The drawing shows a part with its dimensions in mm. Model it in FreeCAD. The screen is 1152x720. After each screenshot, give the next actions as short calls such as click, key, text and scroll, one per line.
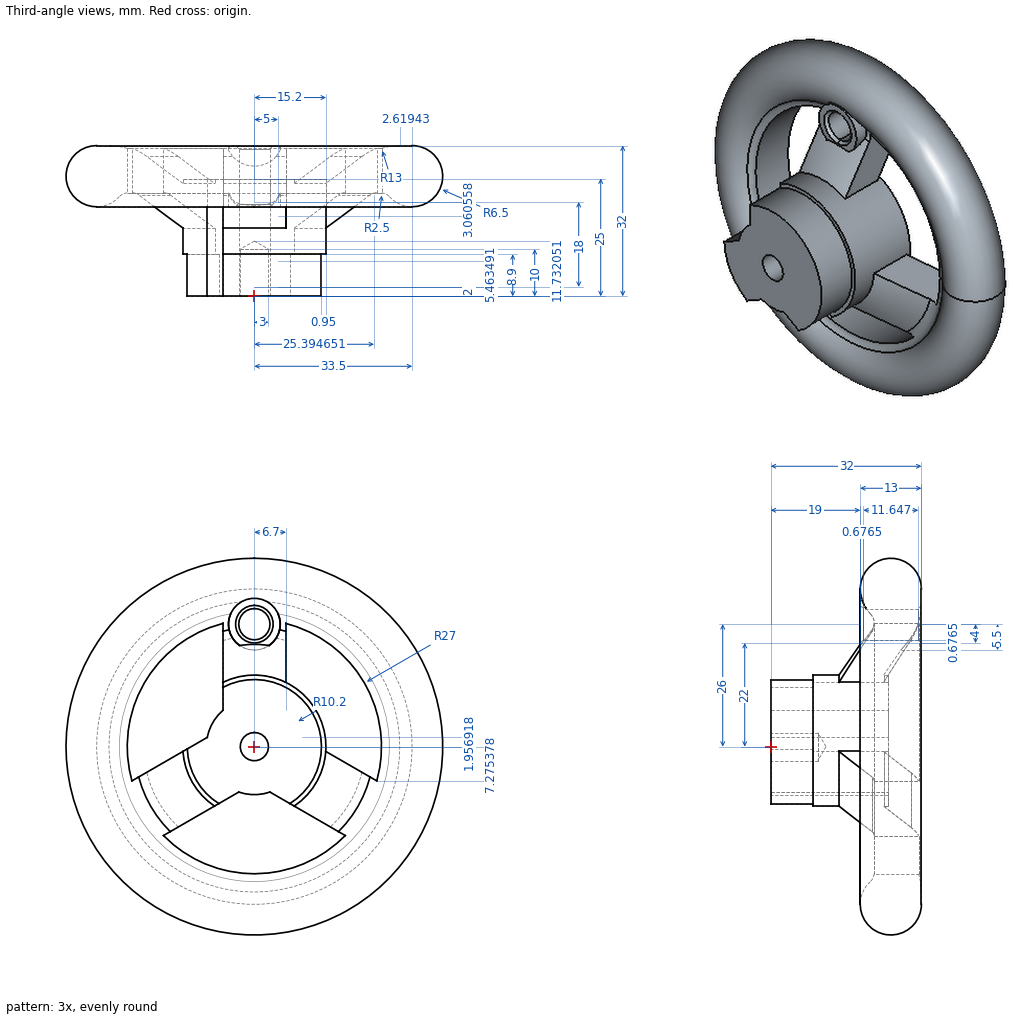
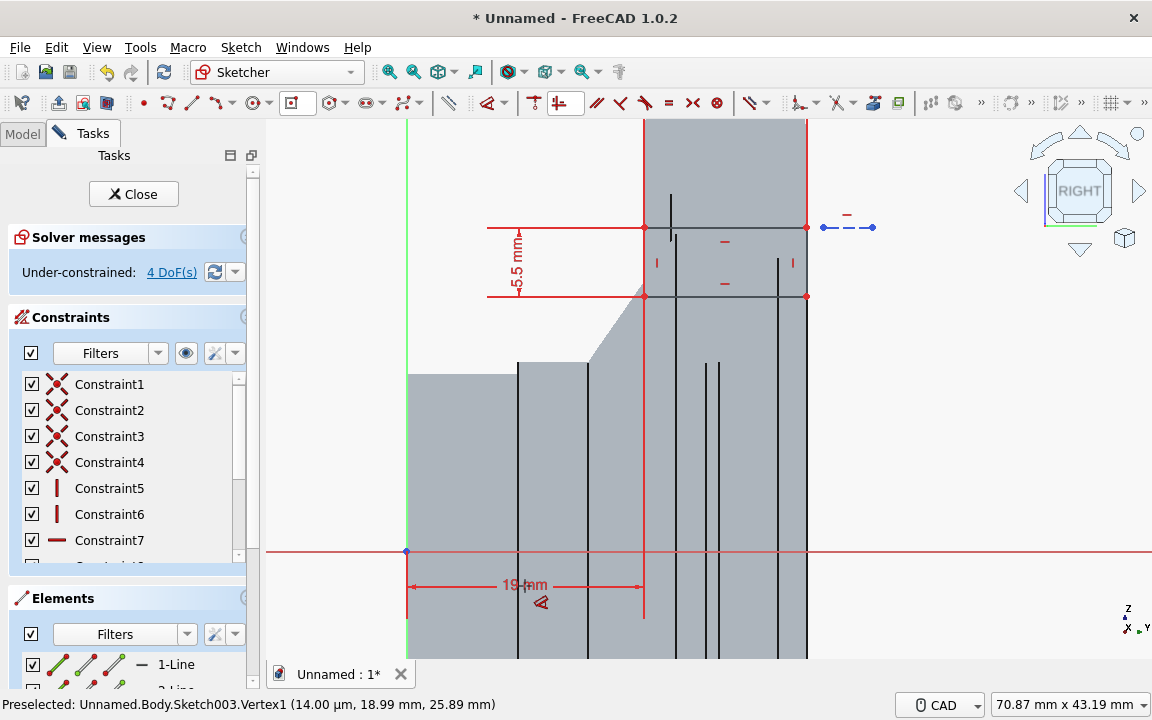
click(644, 228)
click(373, 390)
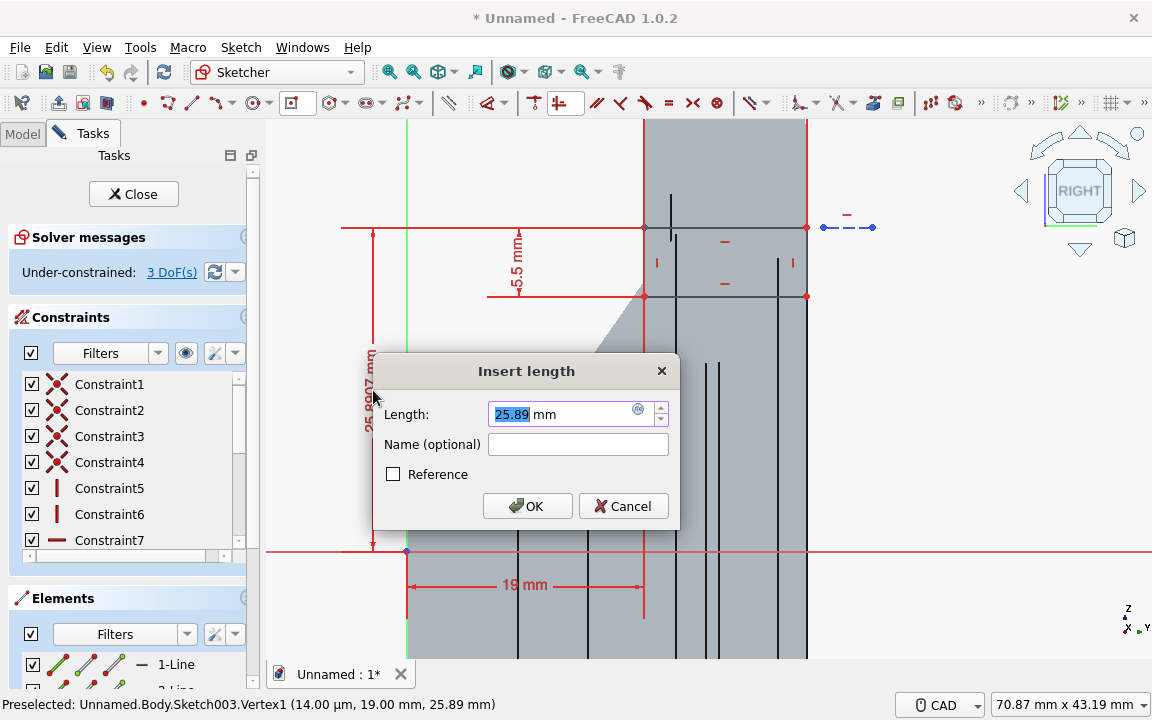
text(26)
key(Return)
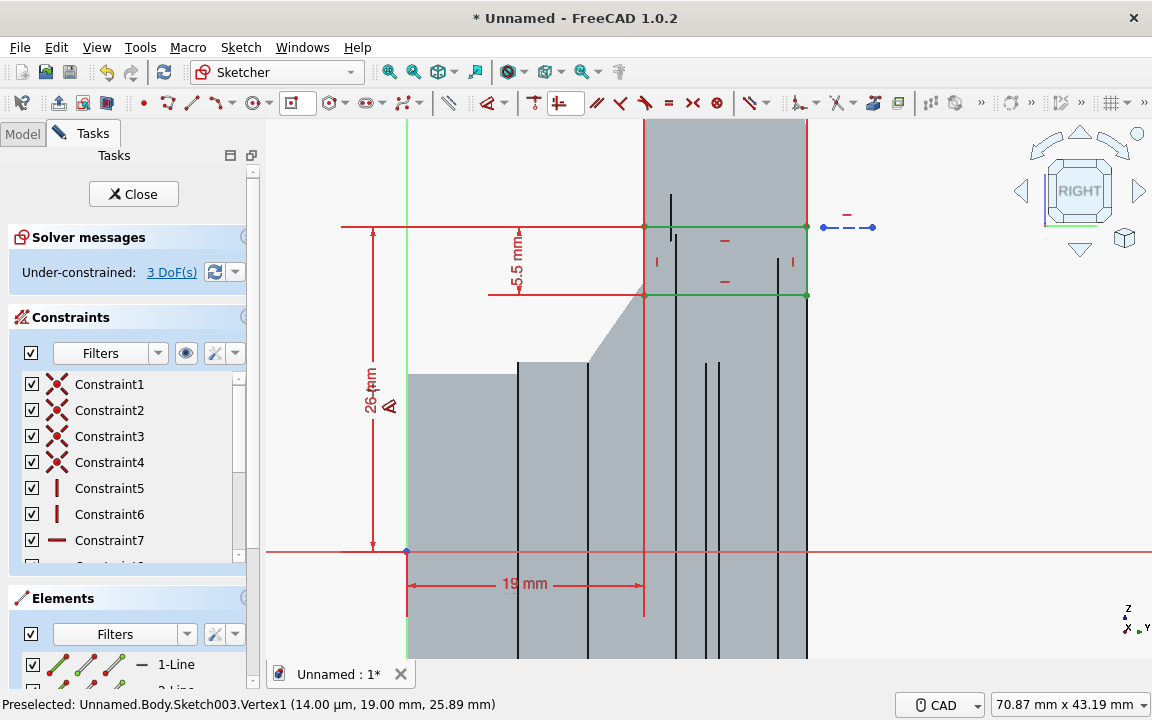
click(823, 228)
click(373, 315)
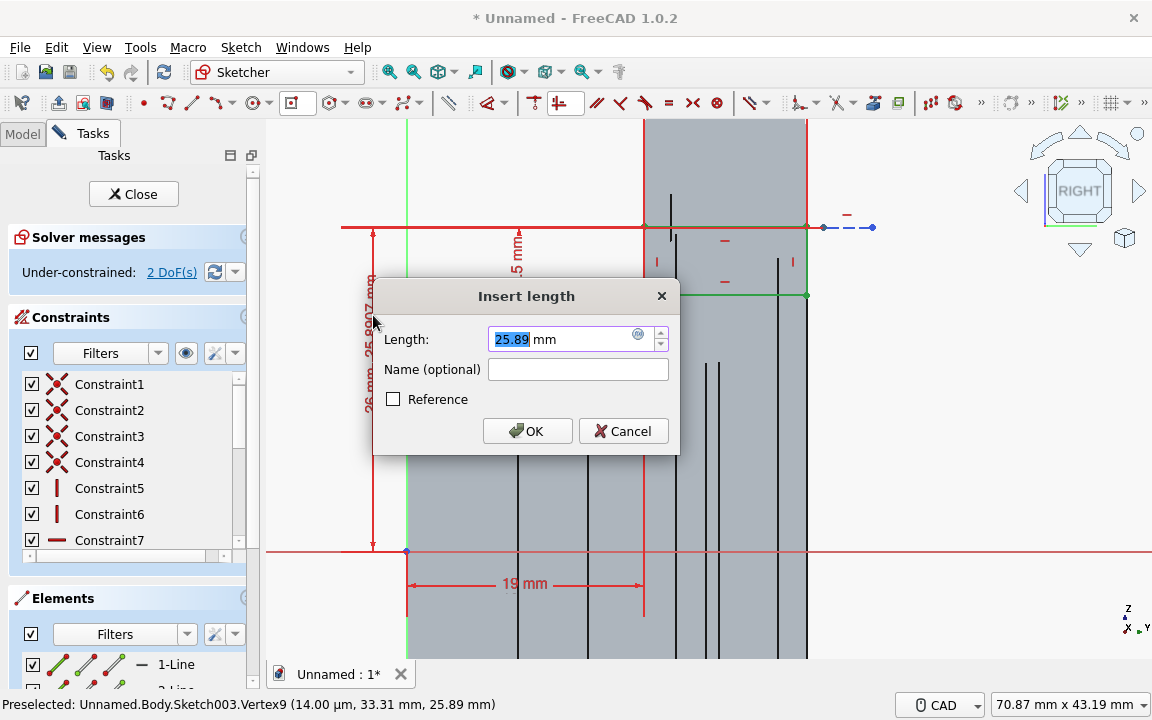
text(26)
key(Return)
key(Escape)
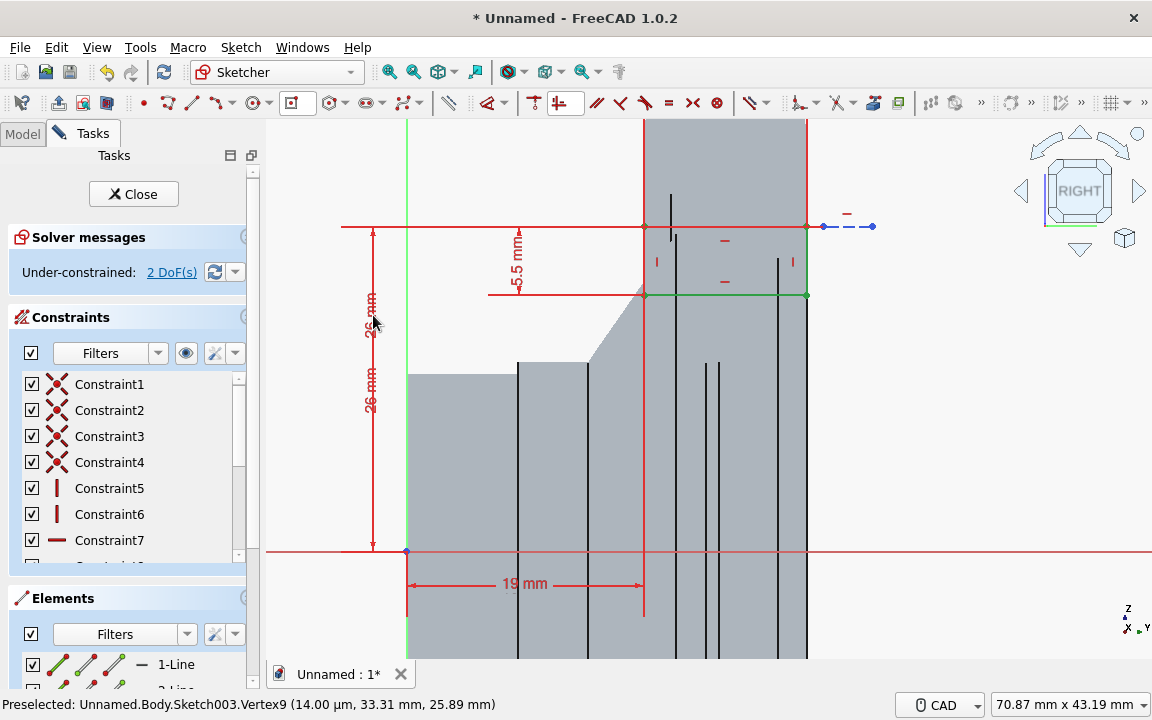
click(134, 194)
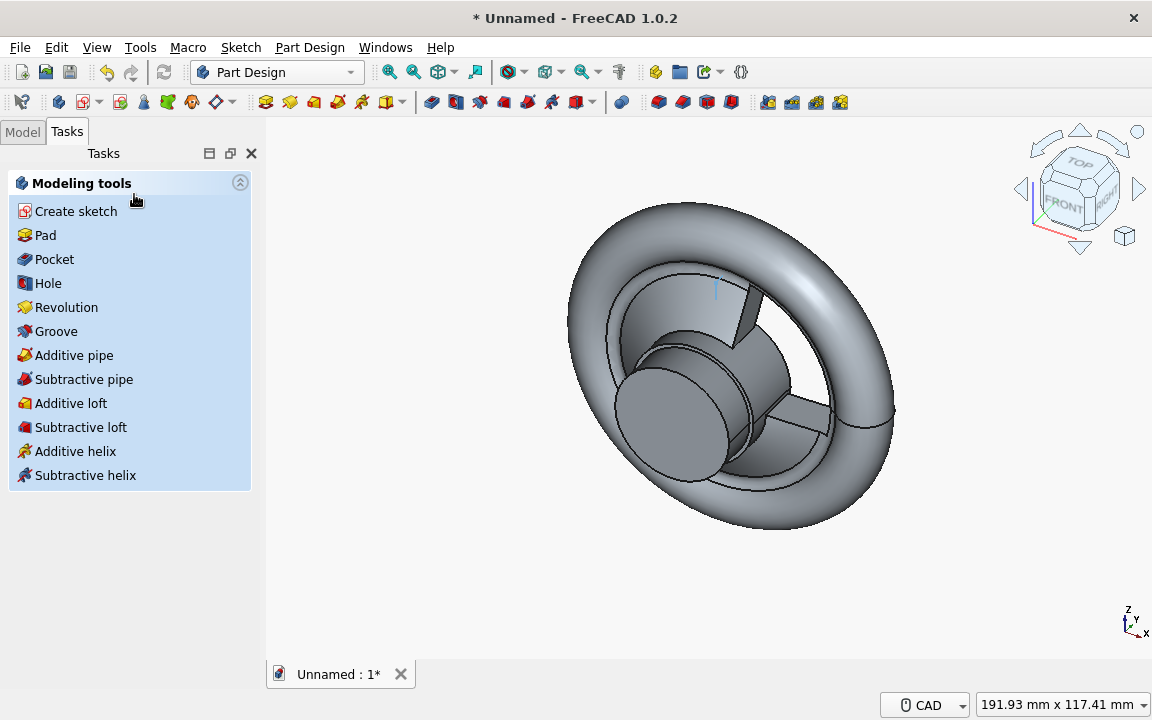
click(290, 102)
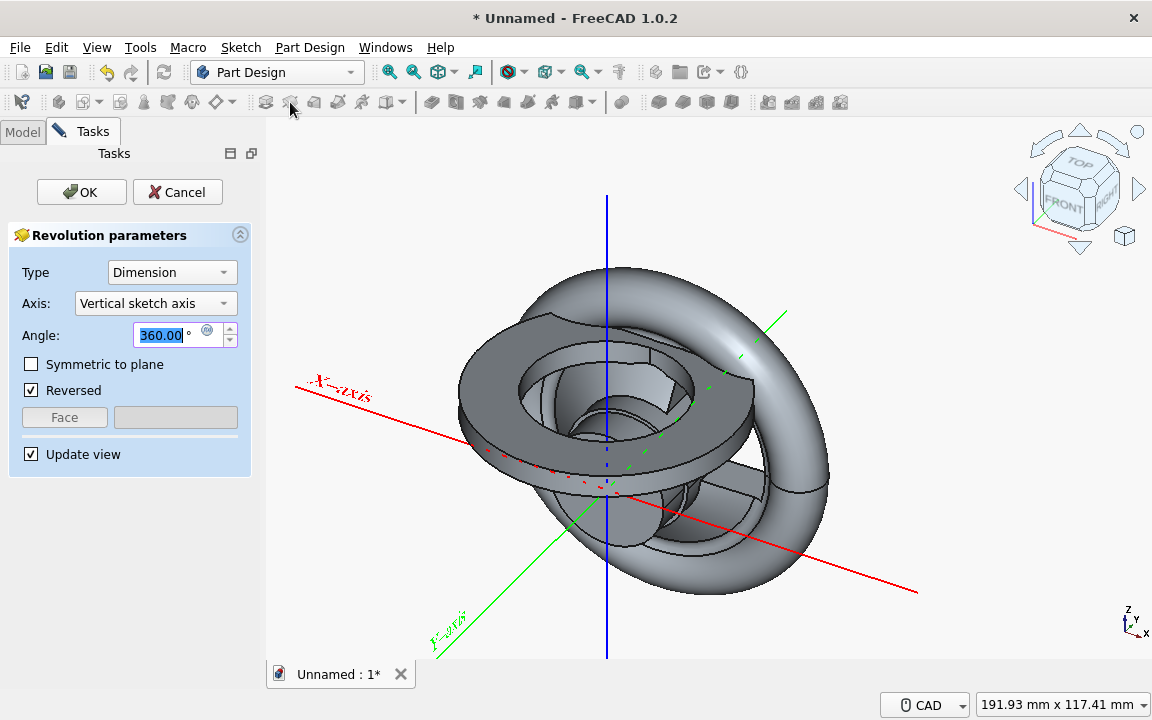
click(156, 304)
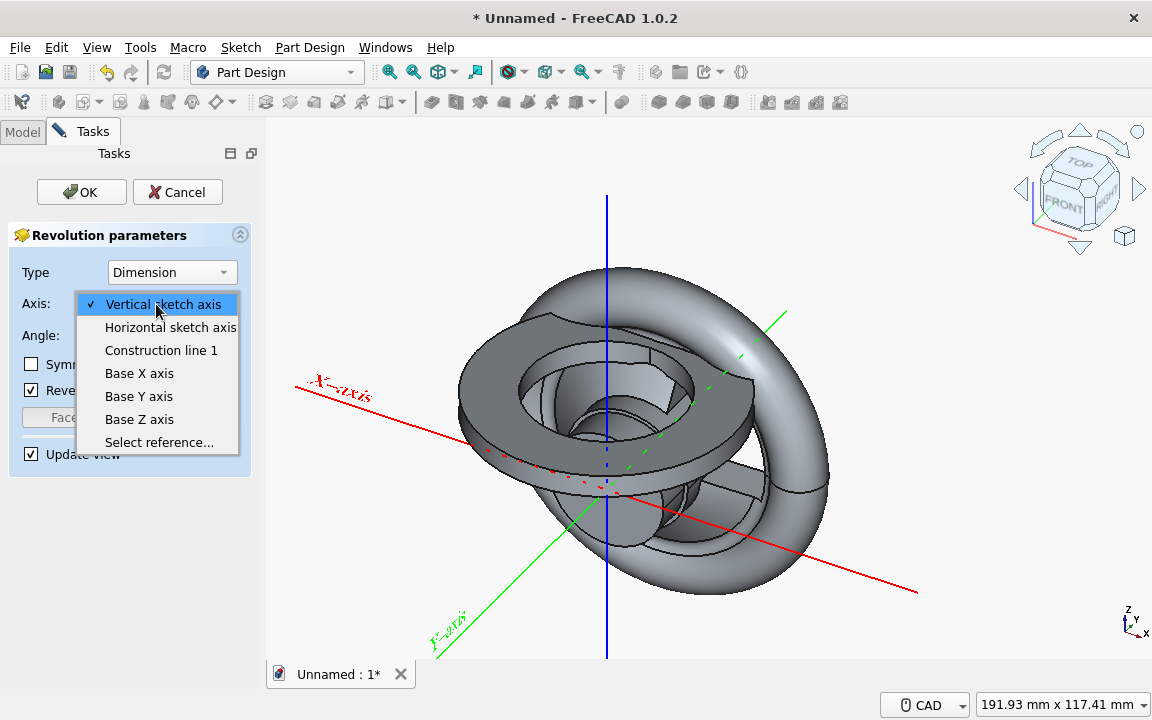
click(156, 350)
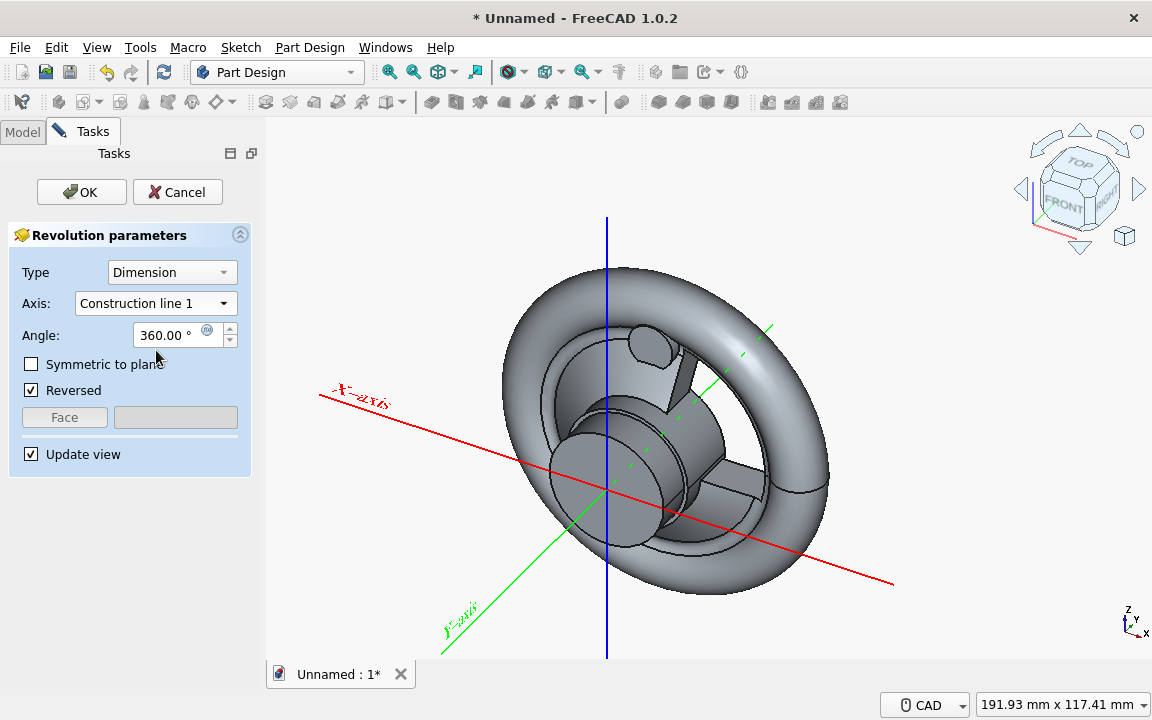
click(82, 192)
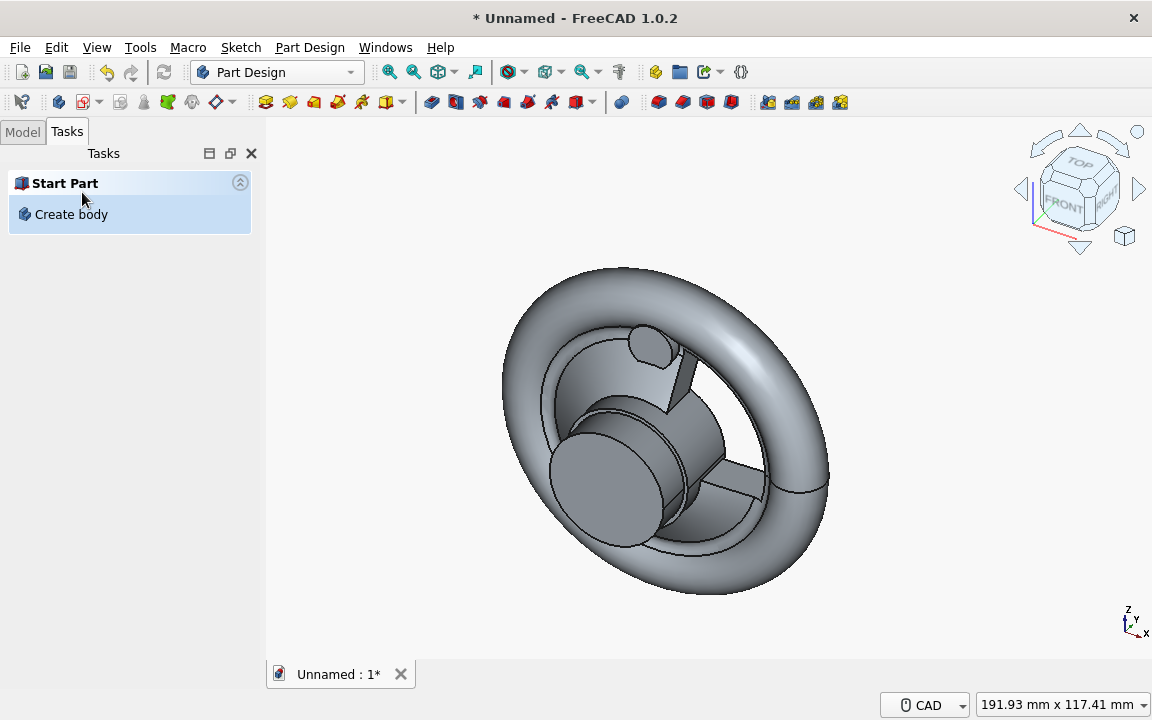
click(390, 72)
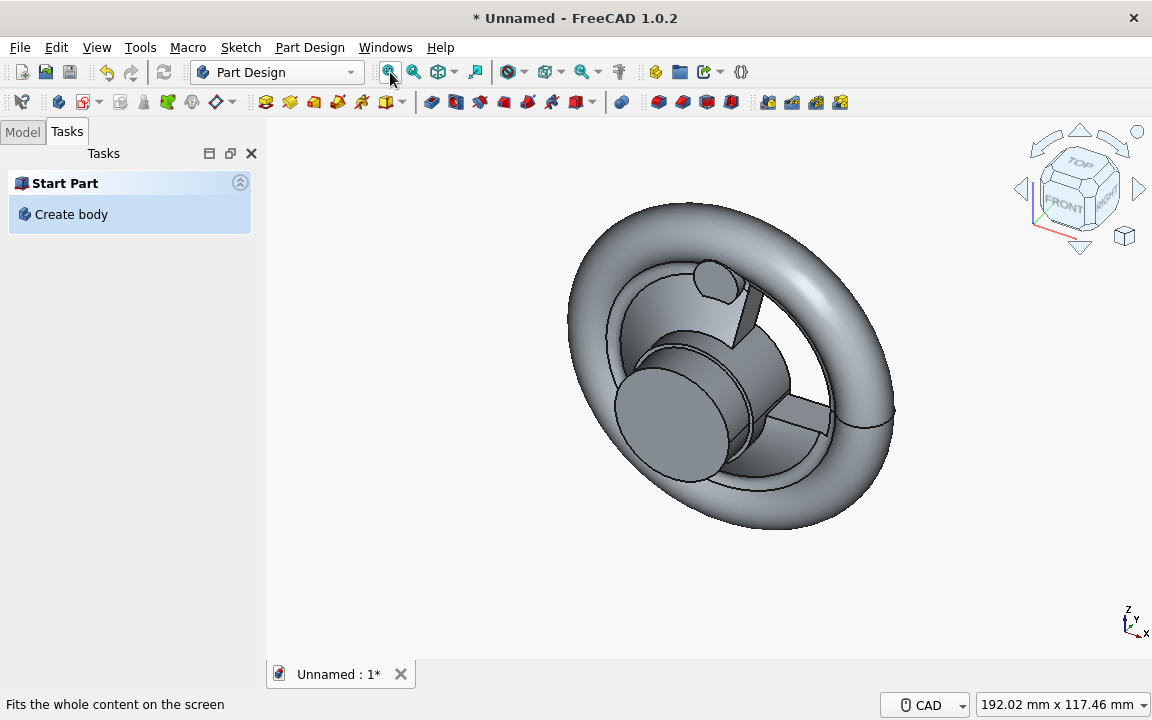
click(84, 102)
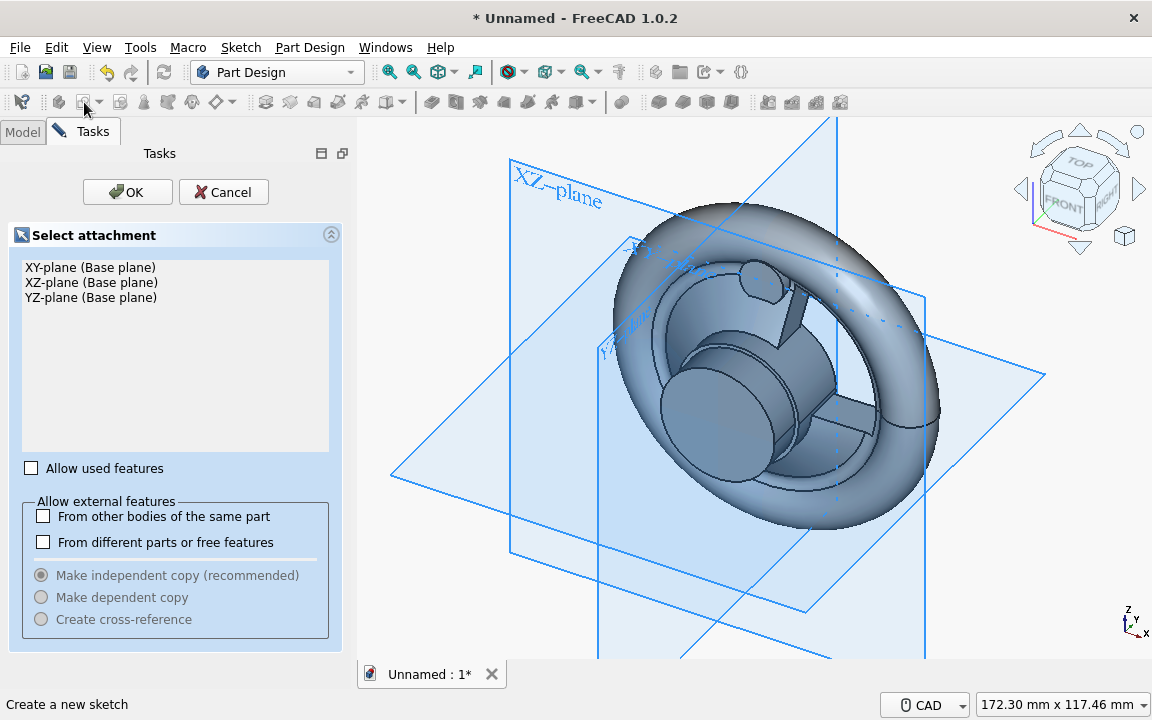
click(82, 298)